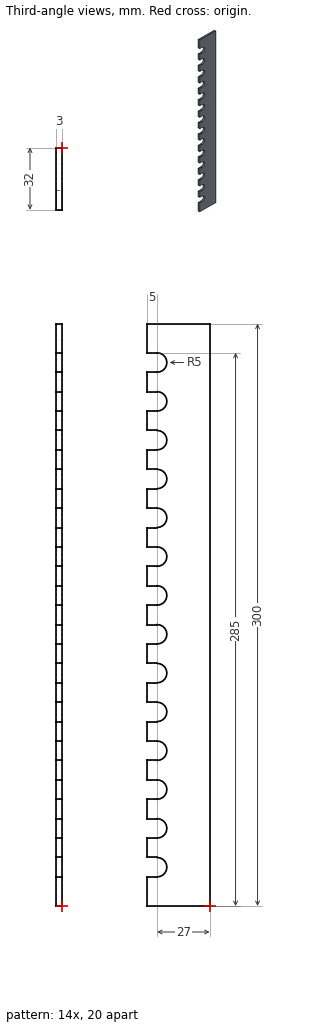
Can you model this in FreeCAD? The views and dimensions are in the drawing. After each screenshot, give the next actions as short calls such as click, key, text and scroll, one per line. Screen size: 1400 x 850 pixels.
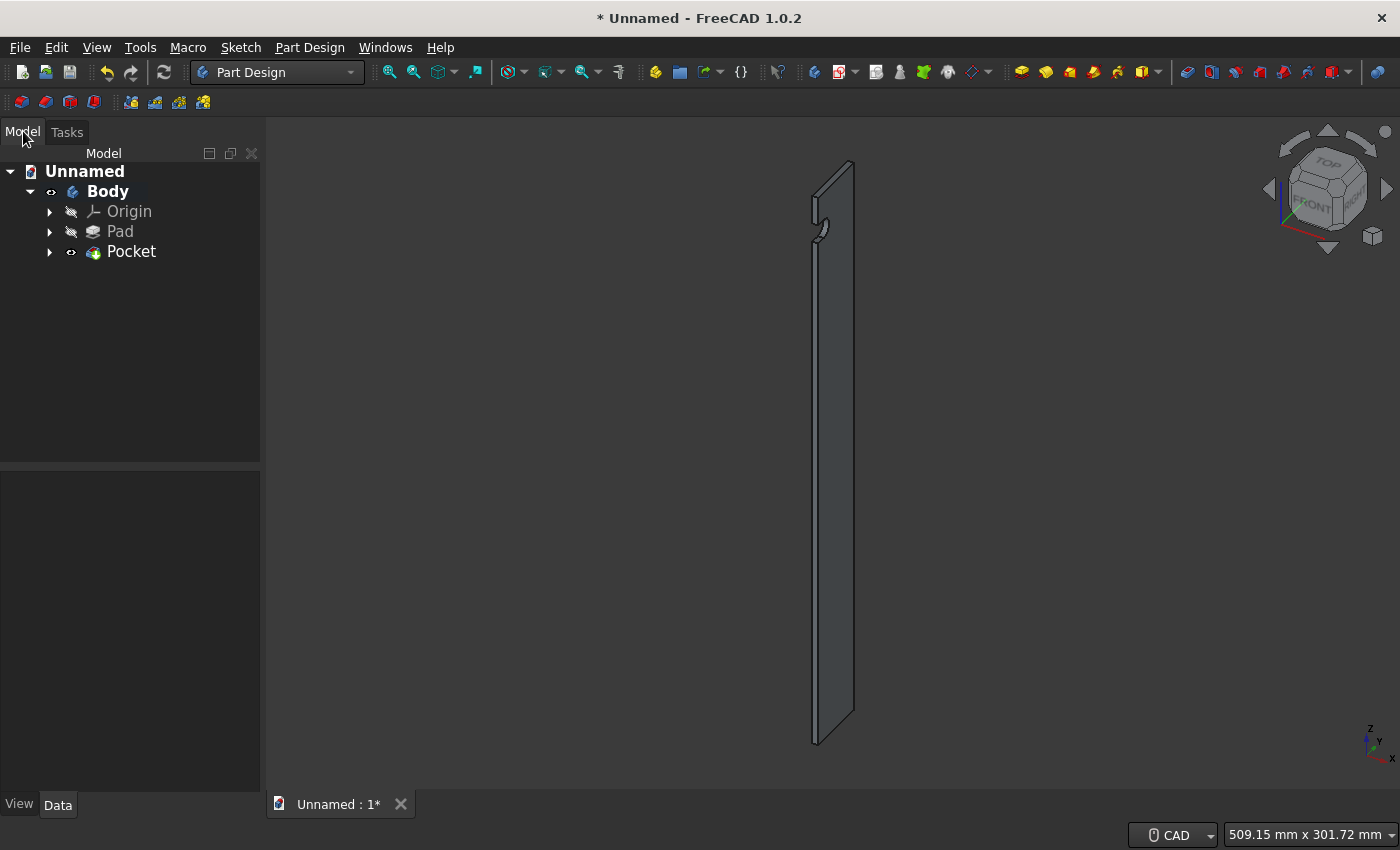
click(116, 252)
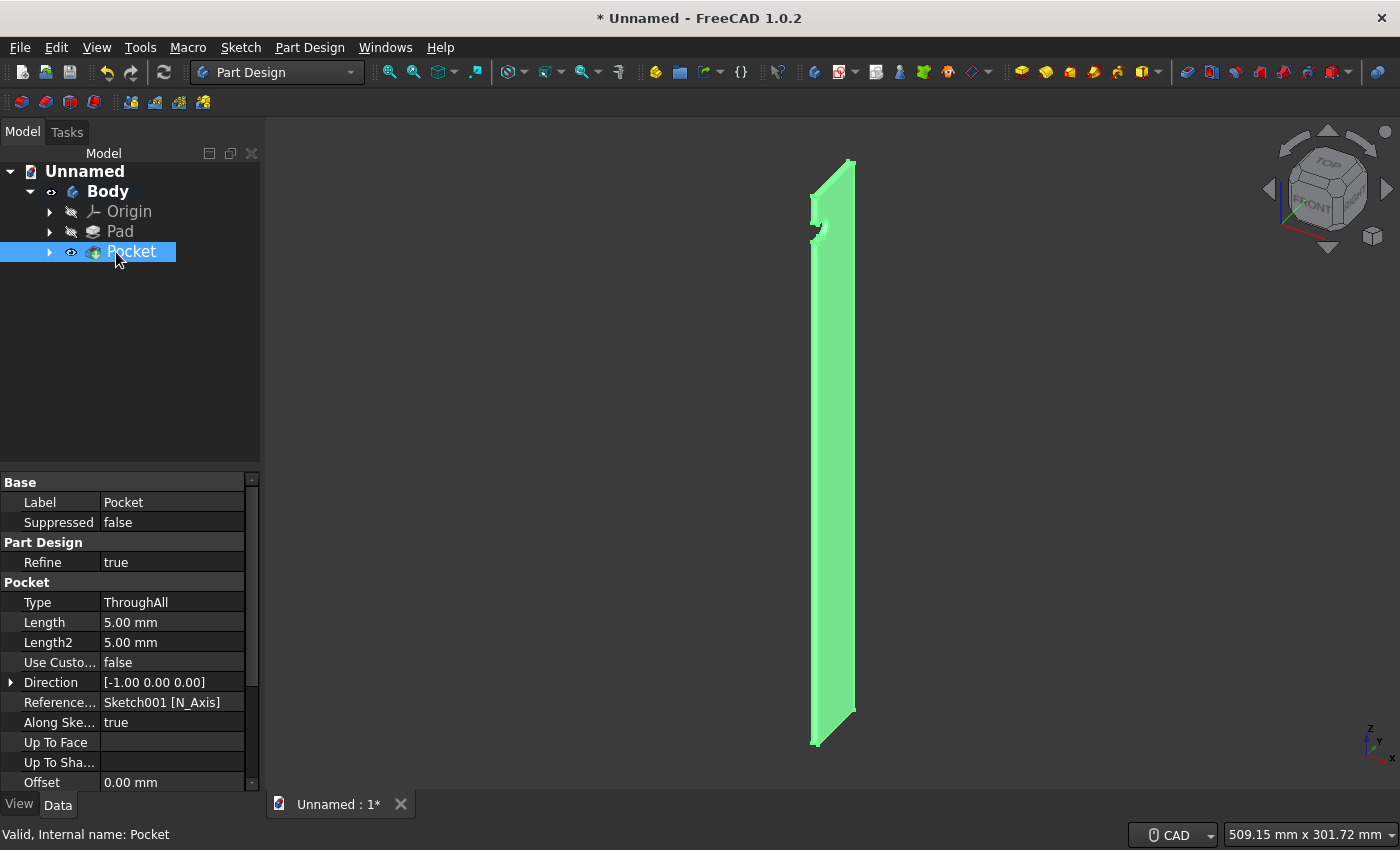
click(156, 102)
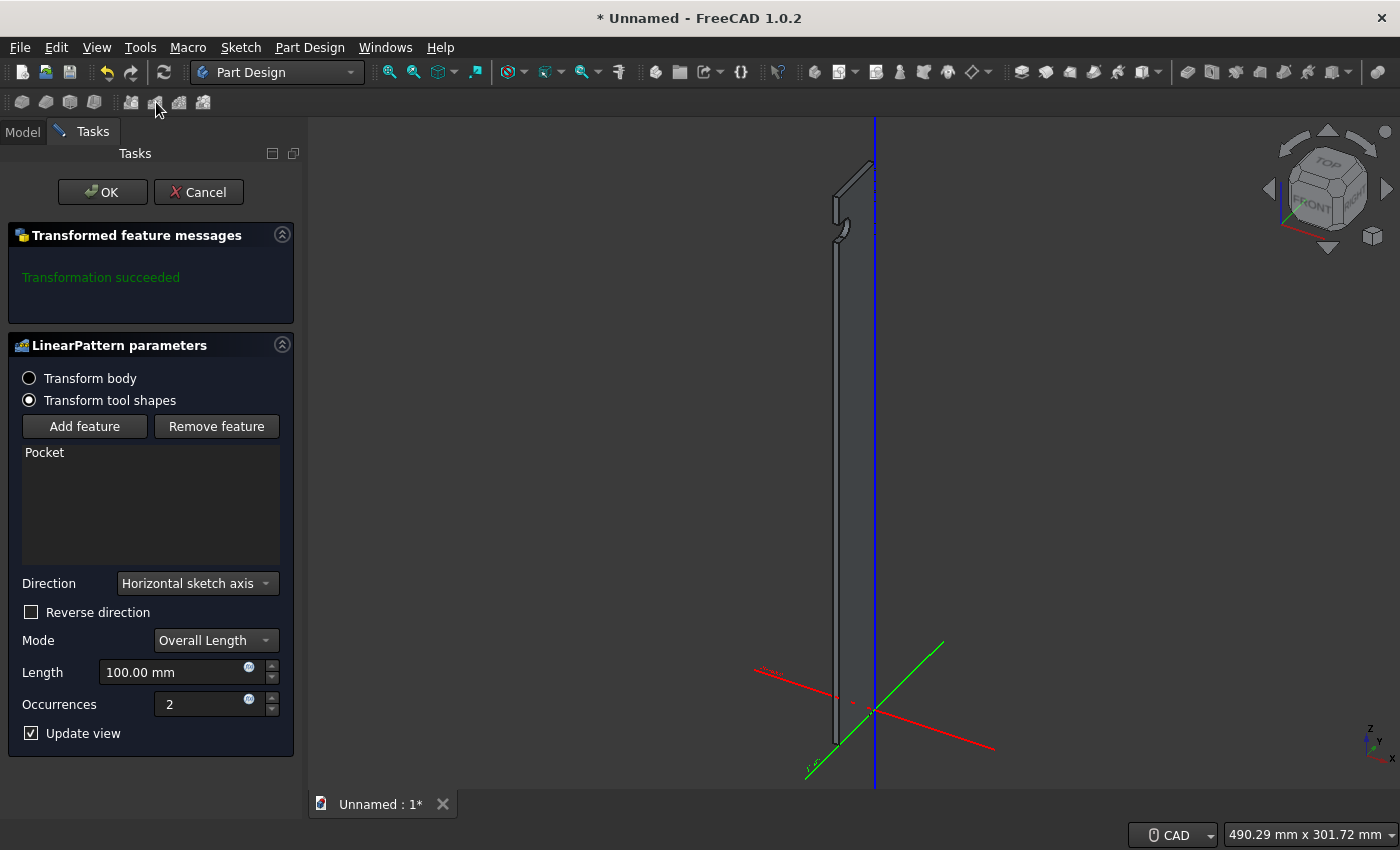
click(198, 584)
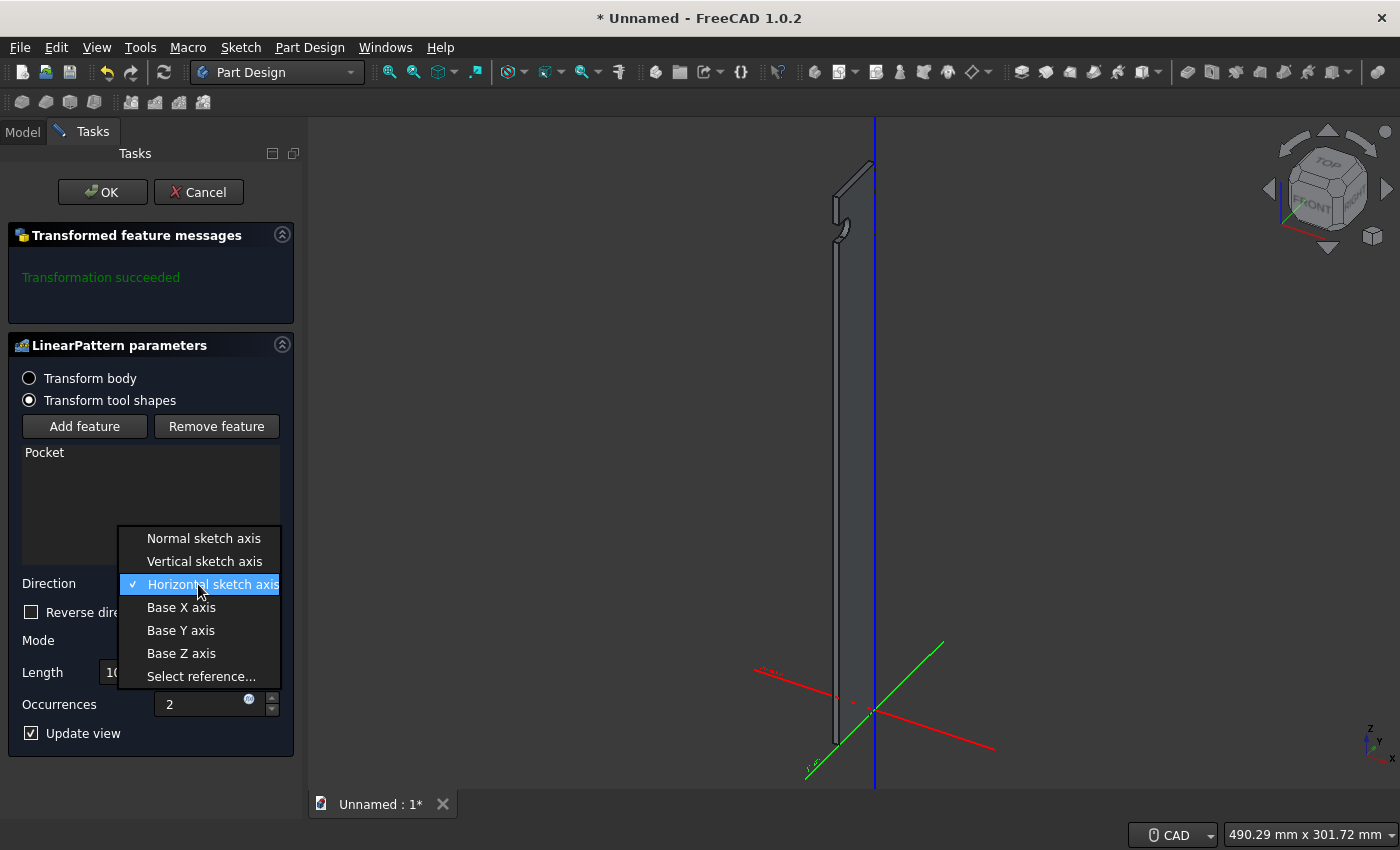
click(198, 654)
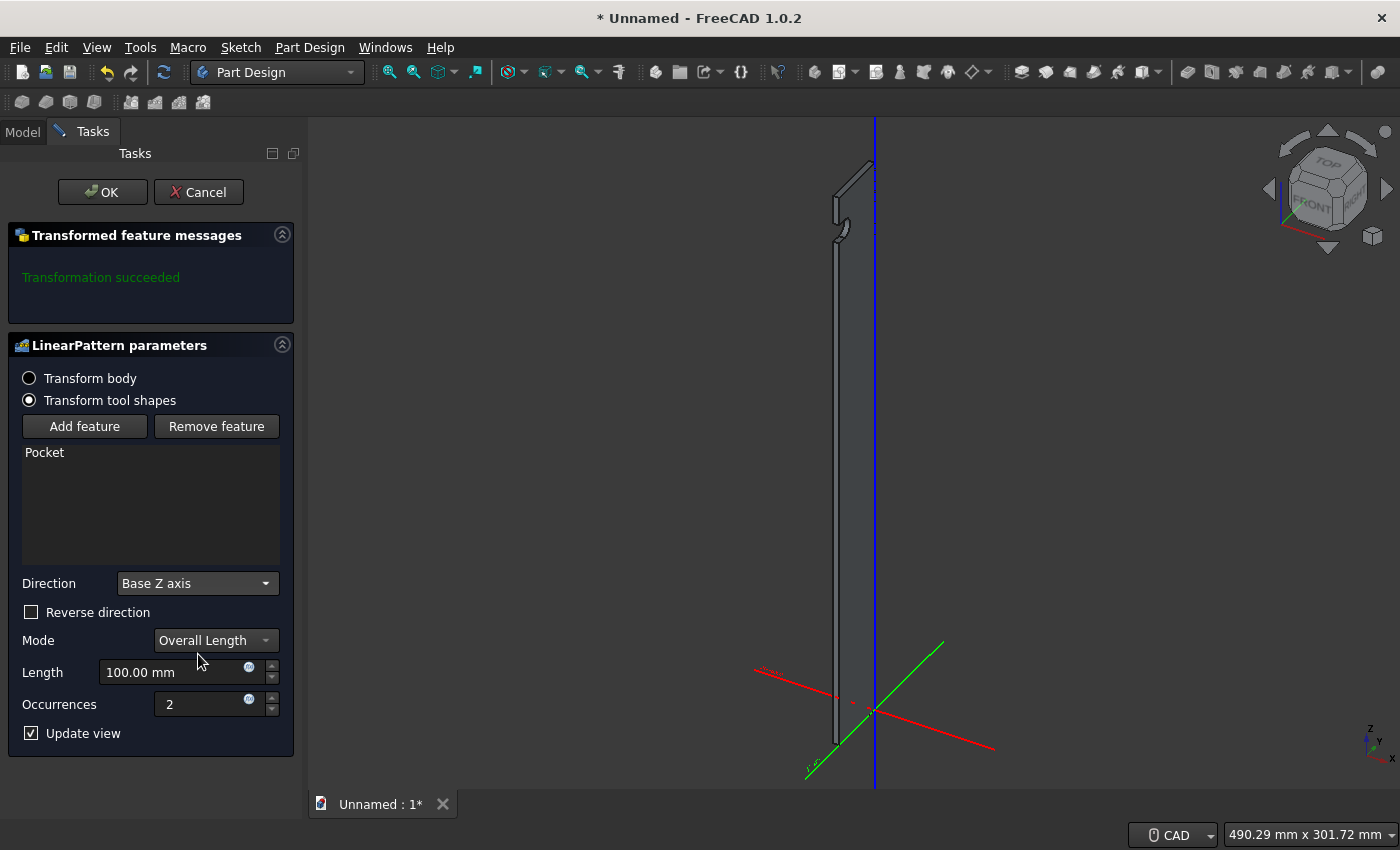
click(217, 640)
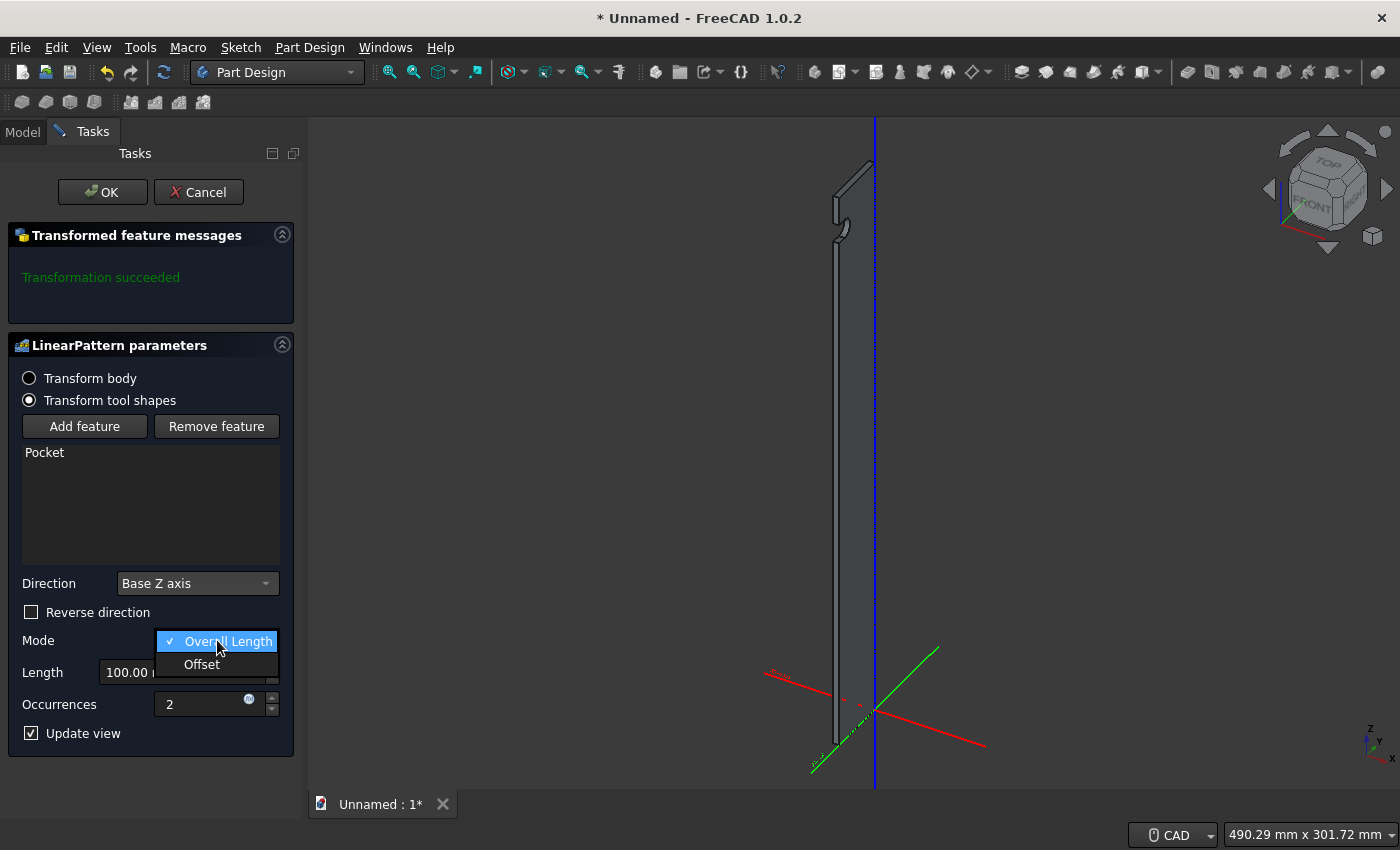
click(216, 664)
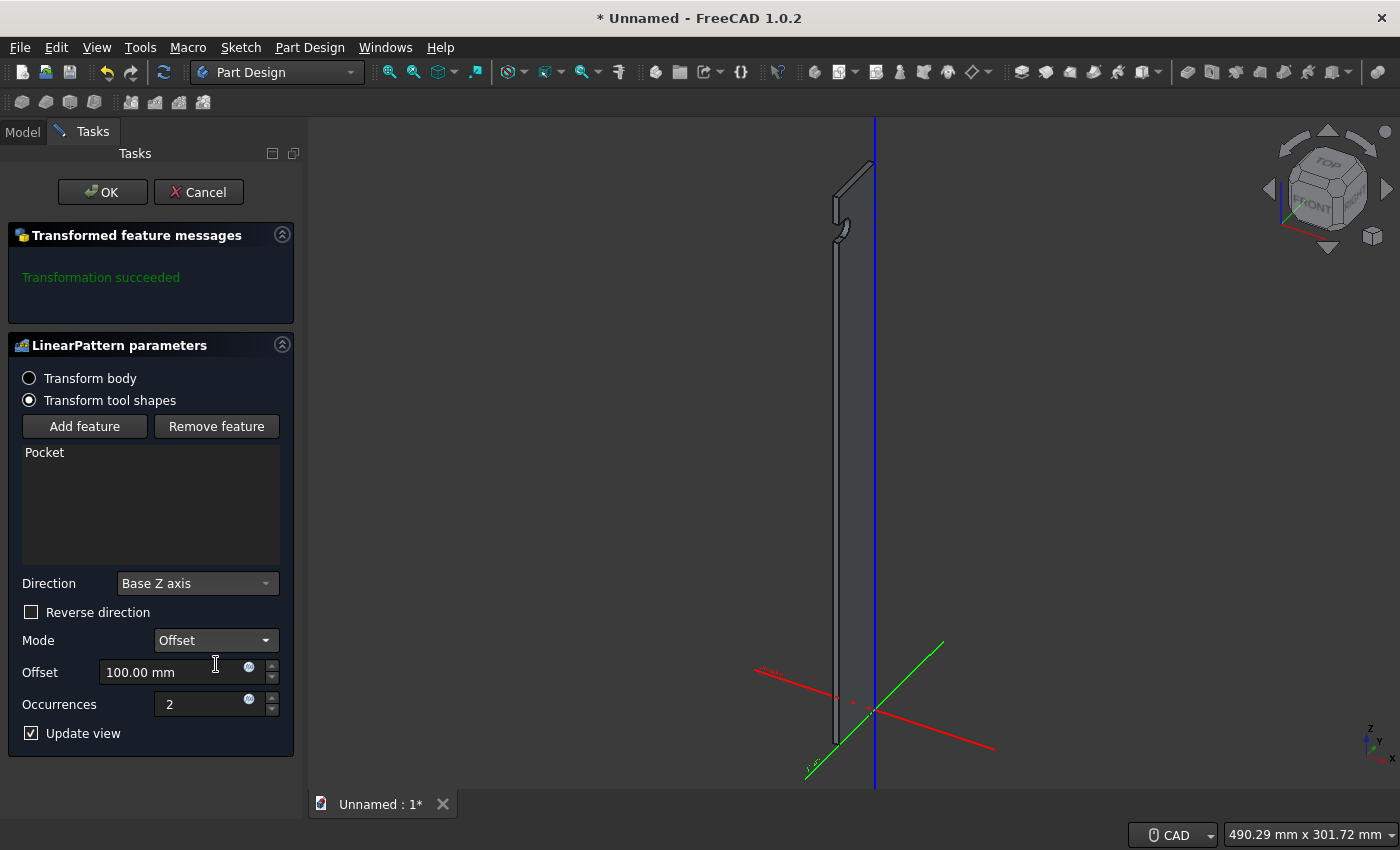
triple_click(182, 672)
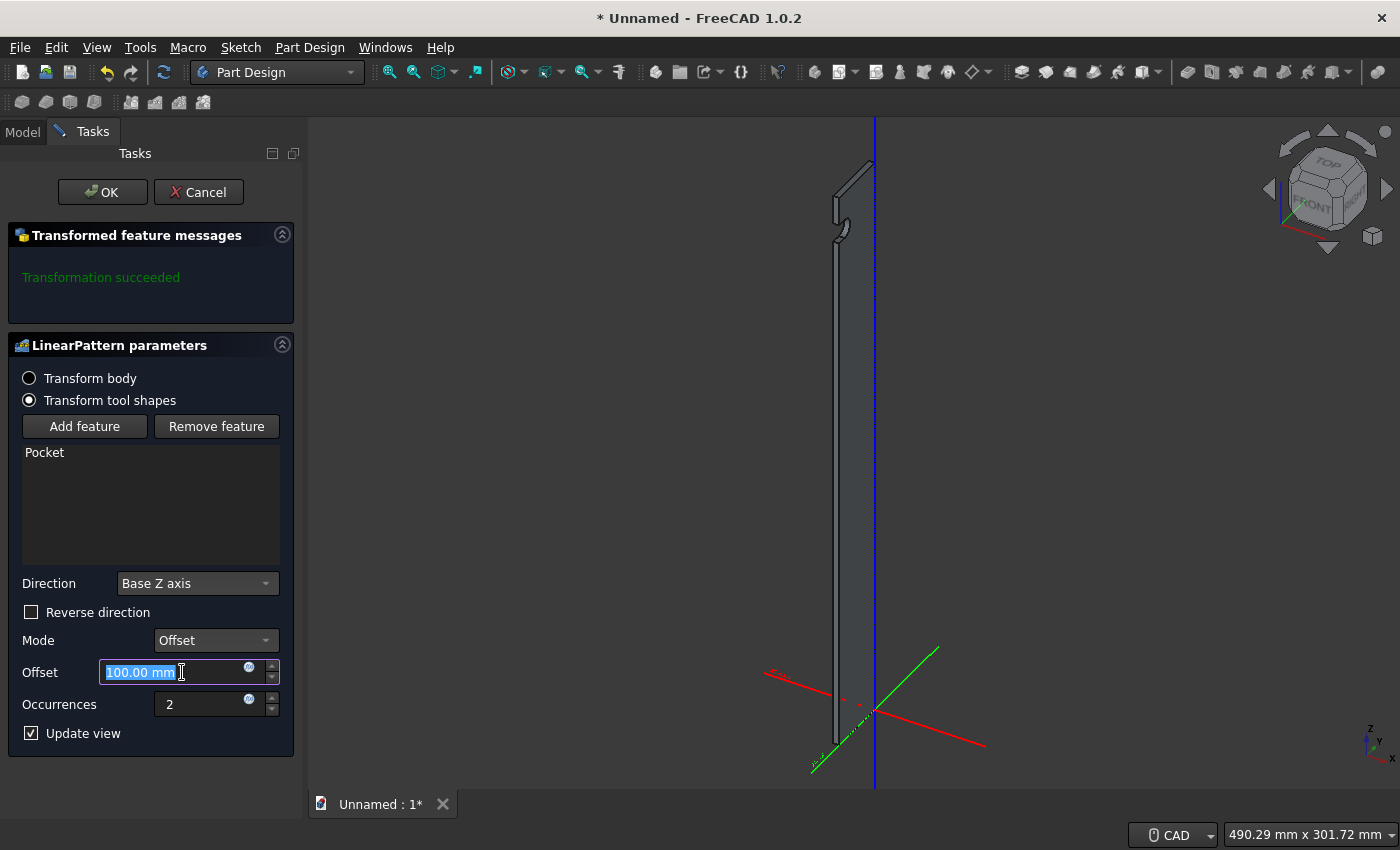
text(20)
key(Tab)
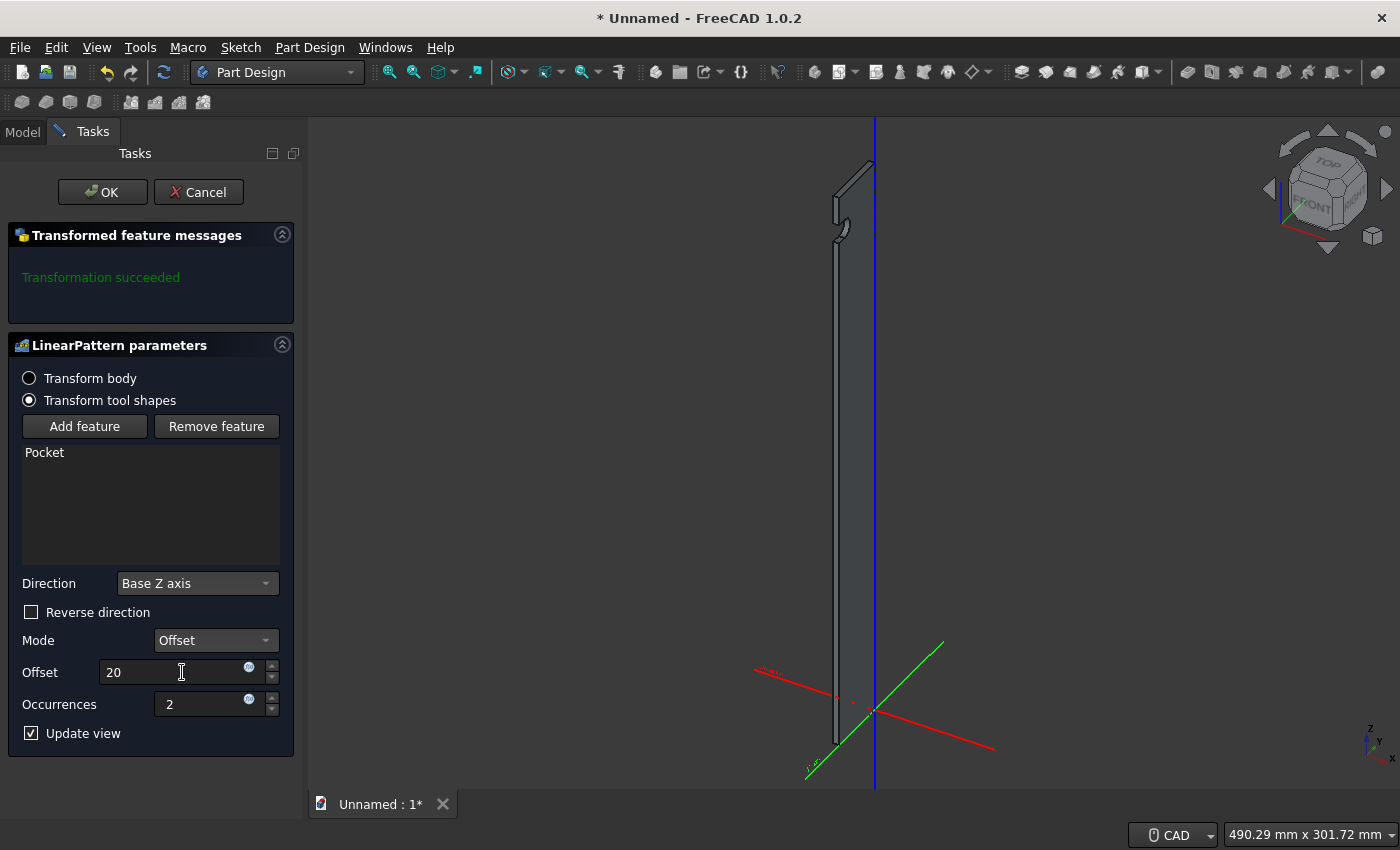
triple_click(209, 704)